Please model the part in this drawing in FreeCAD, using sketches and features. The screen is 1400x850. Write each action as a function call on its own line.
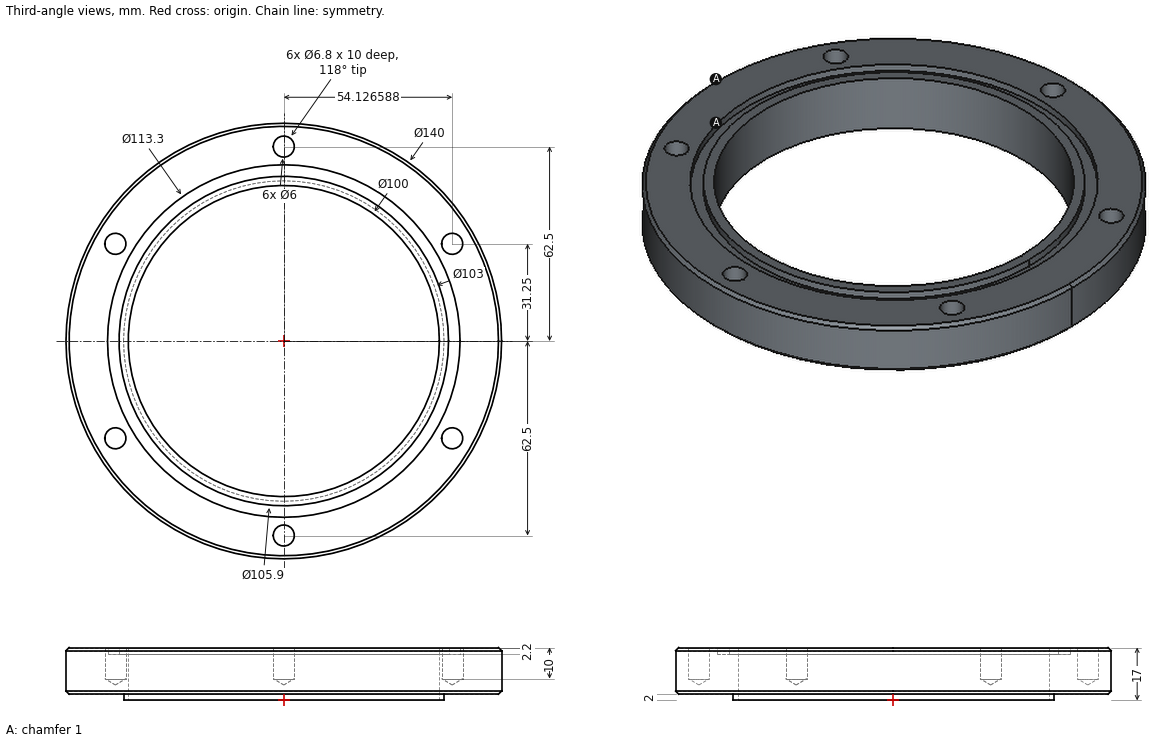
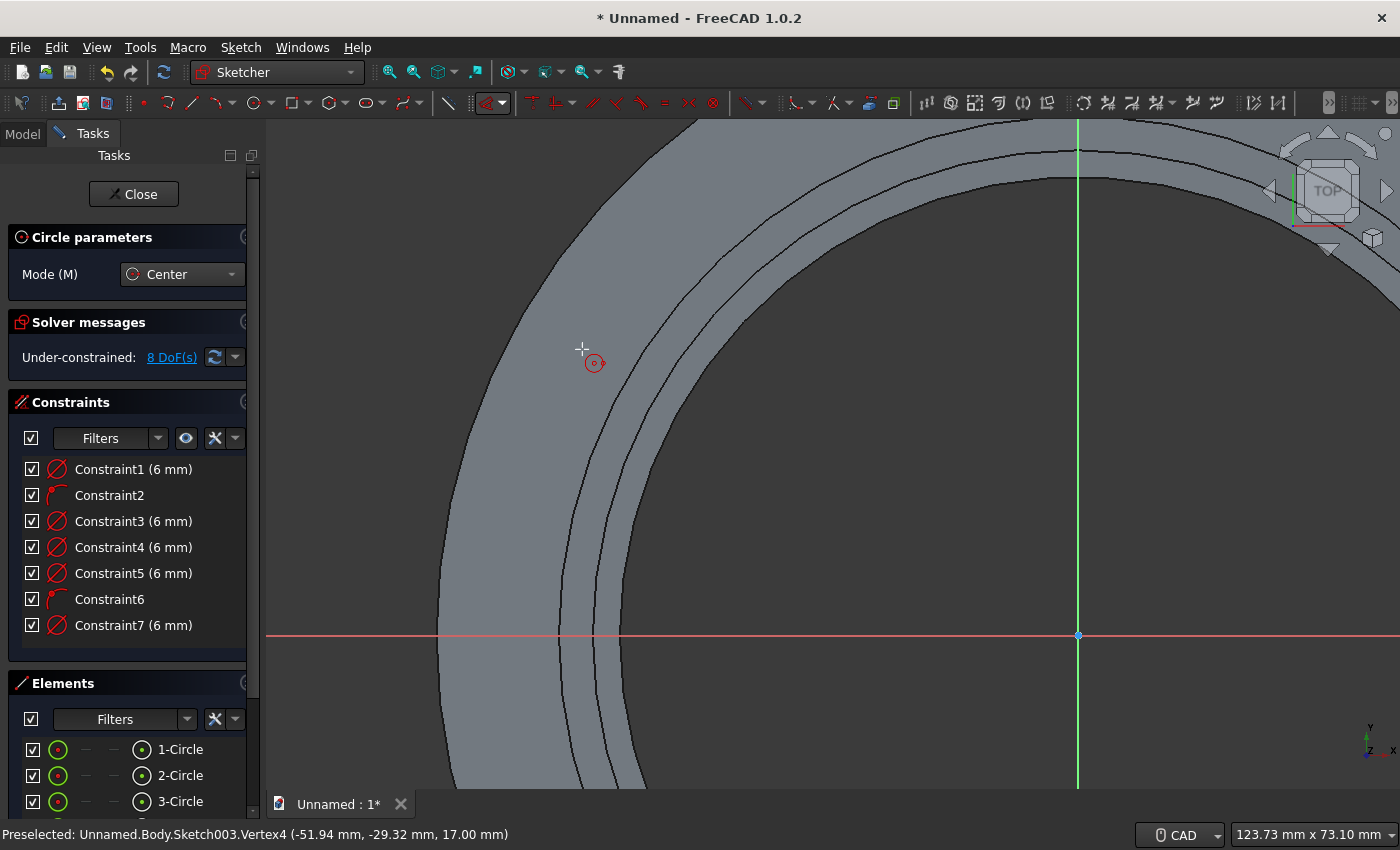
click(582, 349)
move(601, 330)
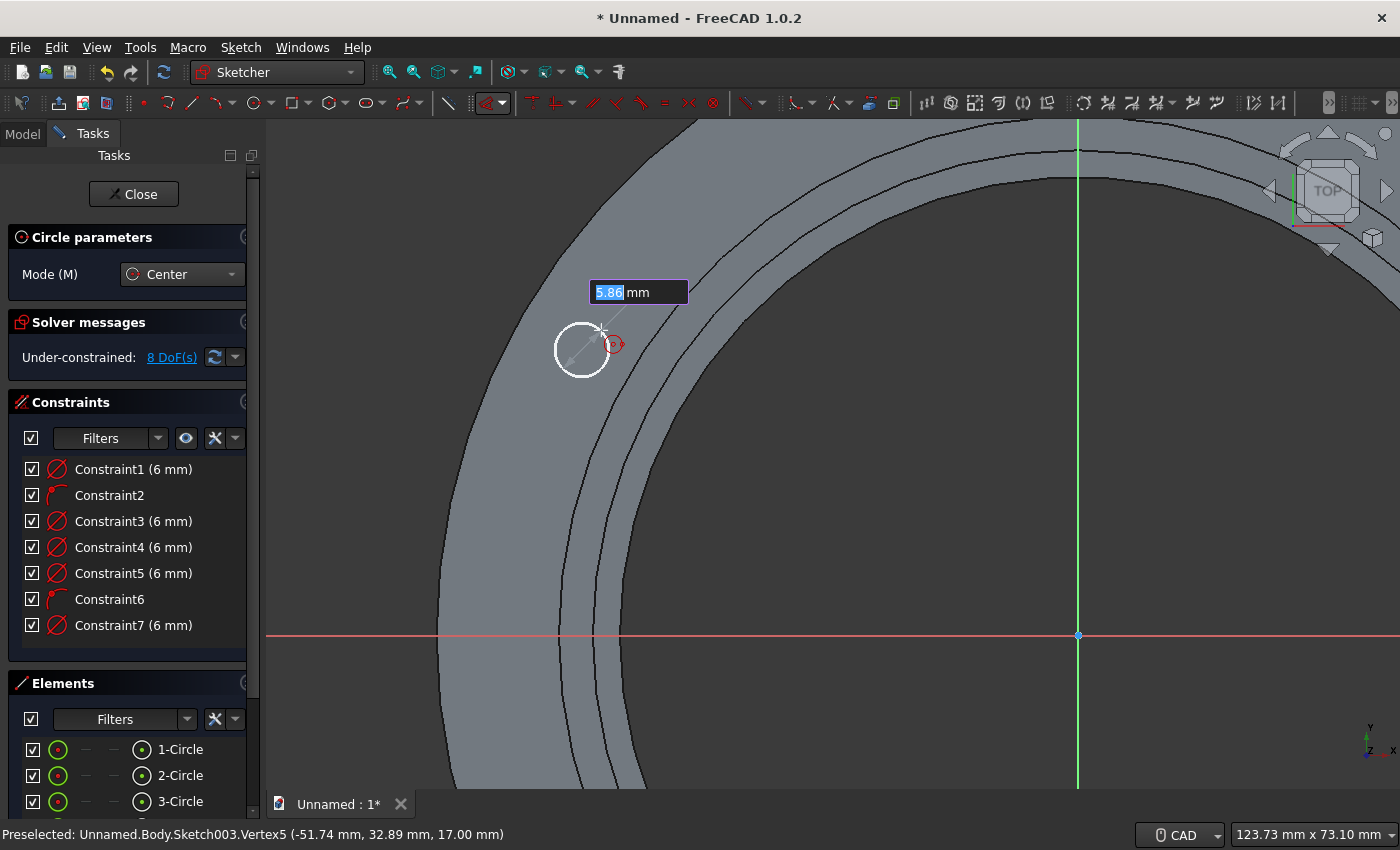
text(6)
key(Return)
key(Escape)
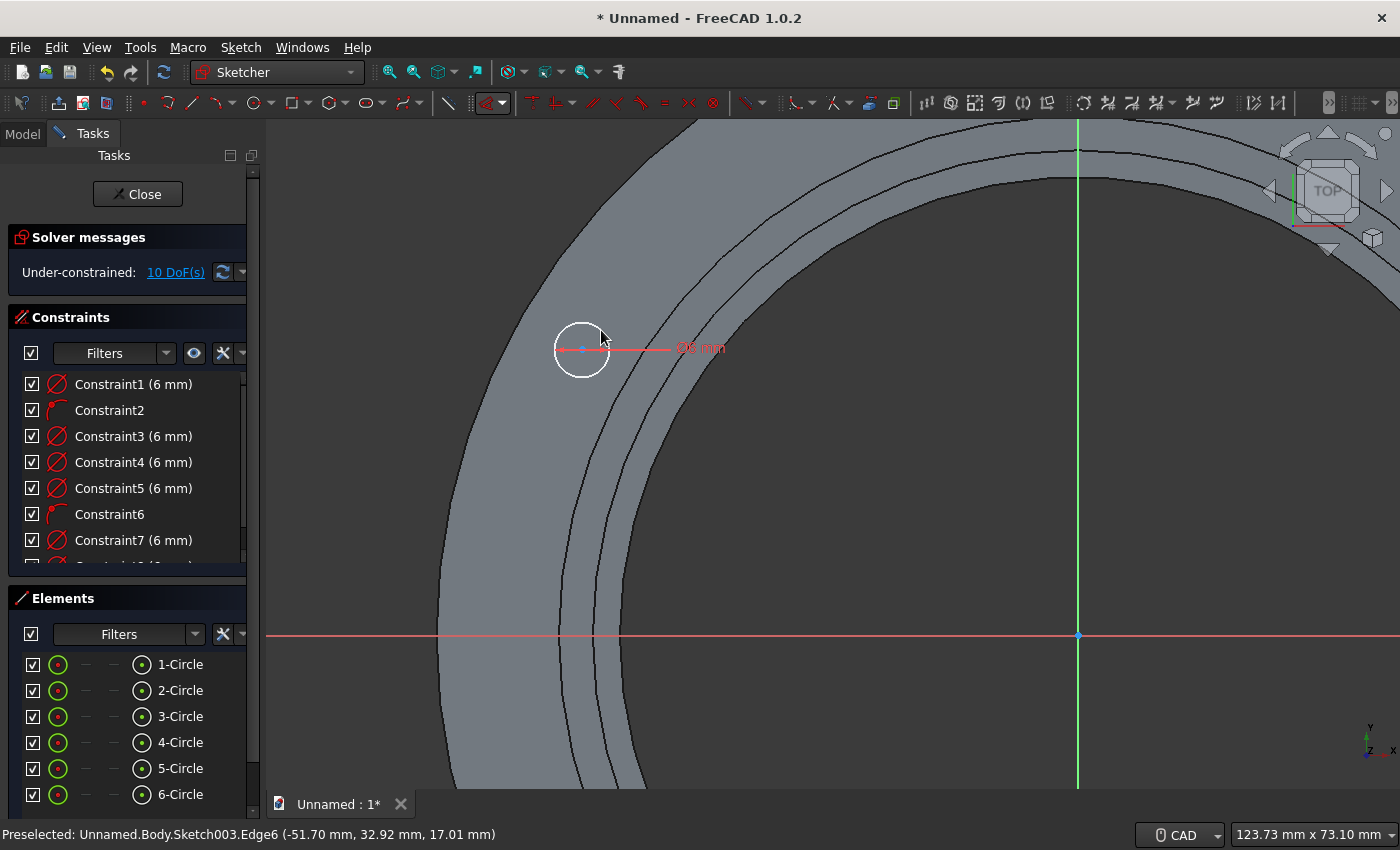
scroll(582, 348, down, 5)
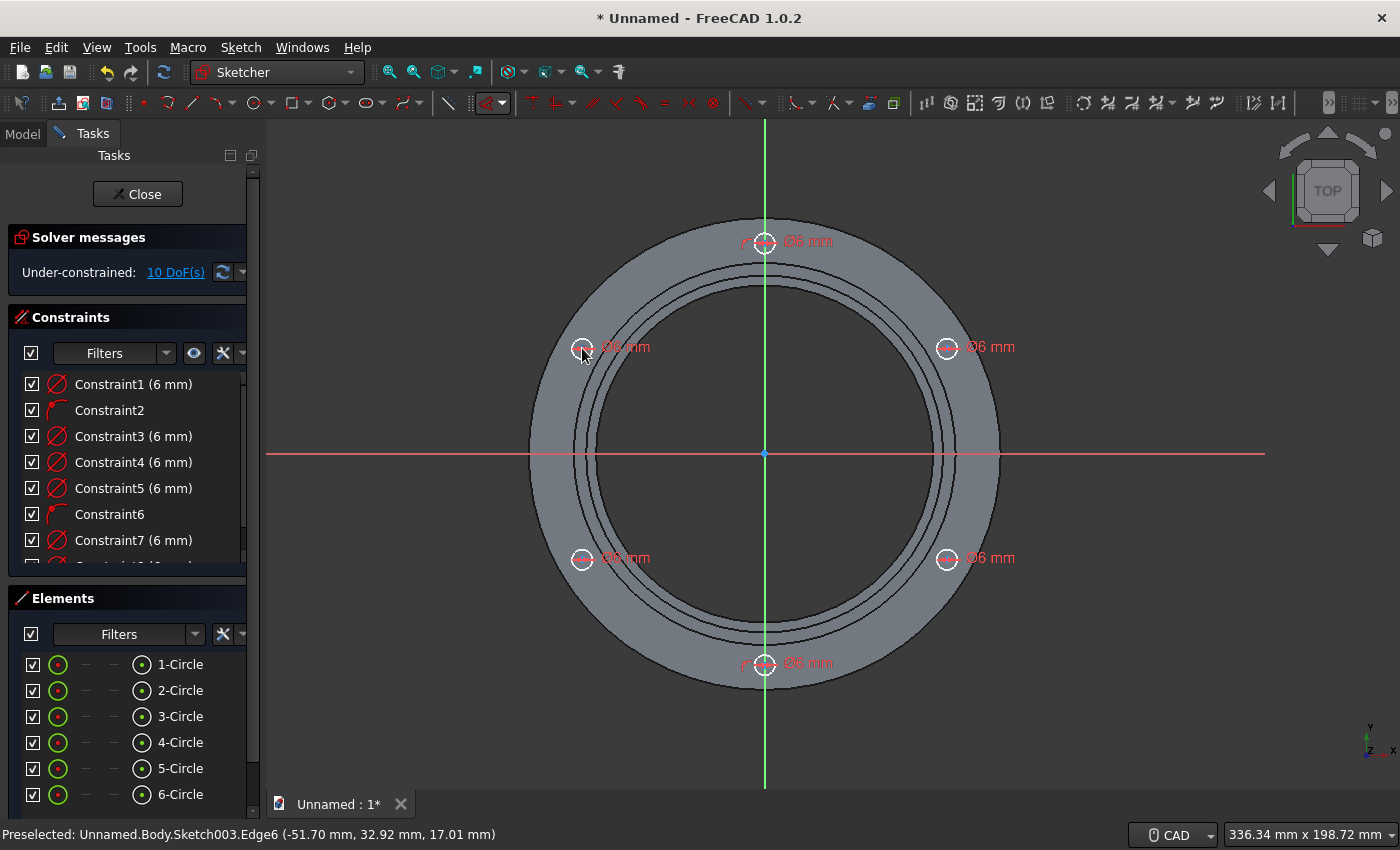
click(947, 349)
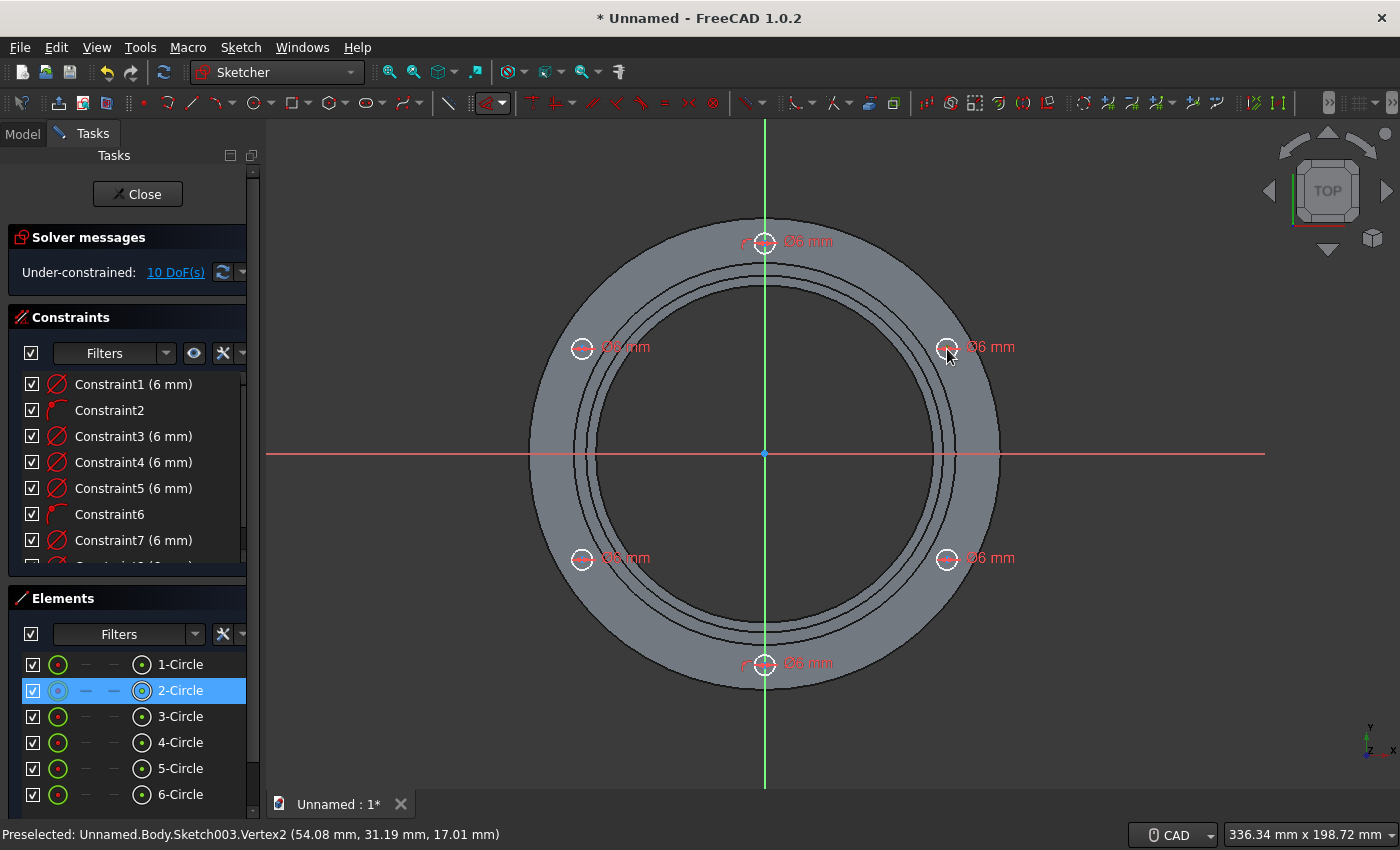
click(947, 560)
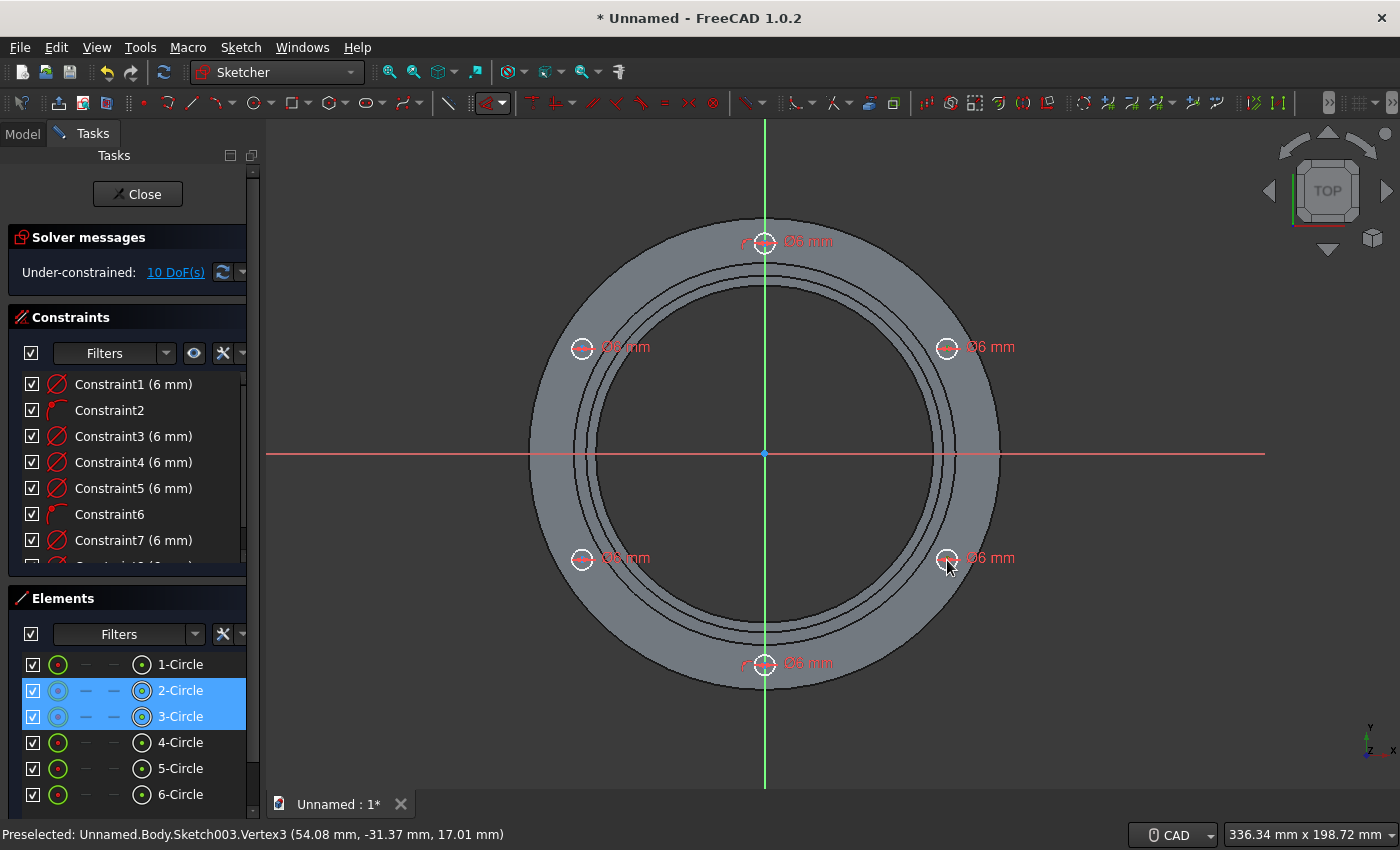
click(361, 454)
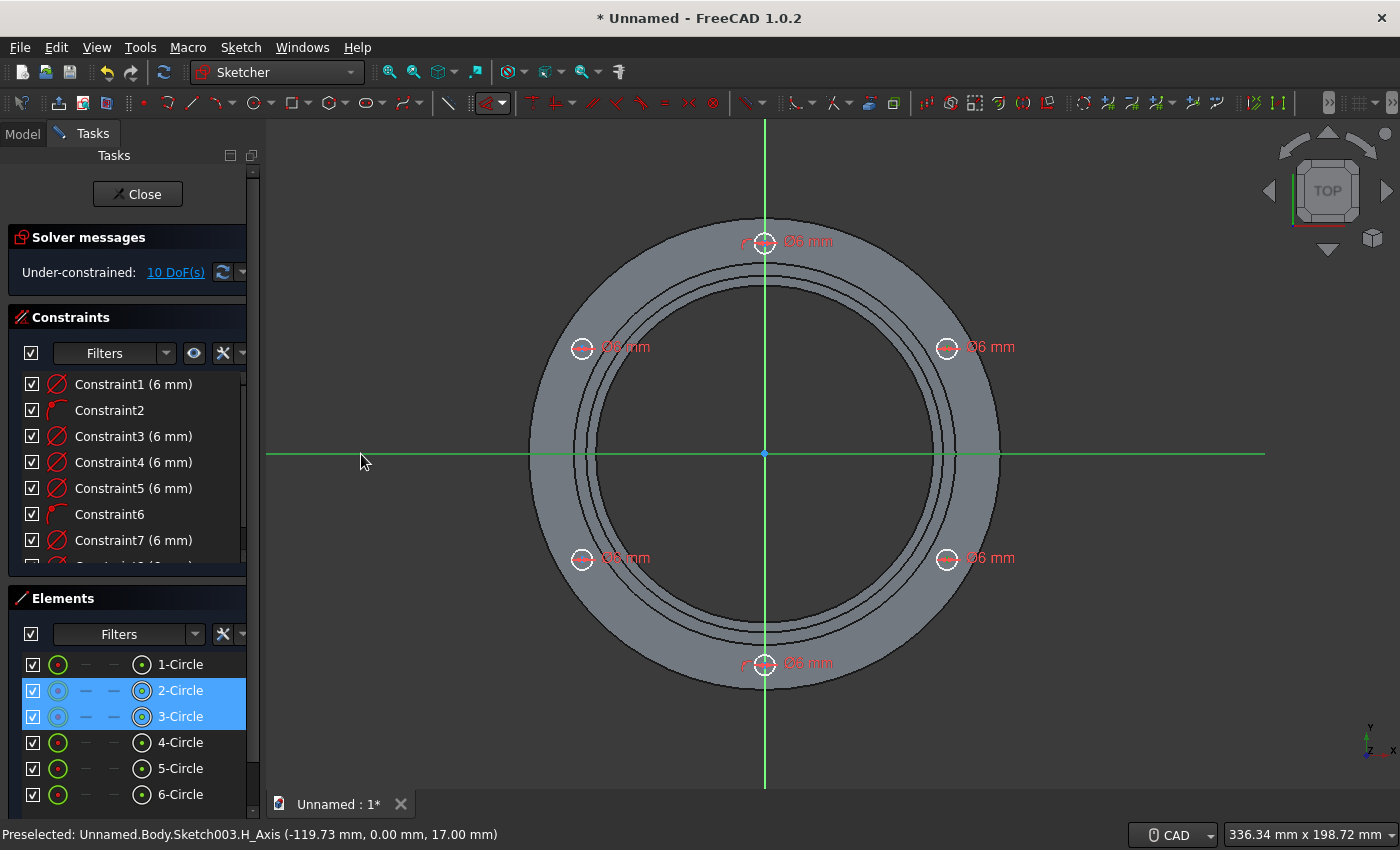
key(s)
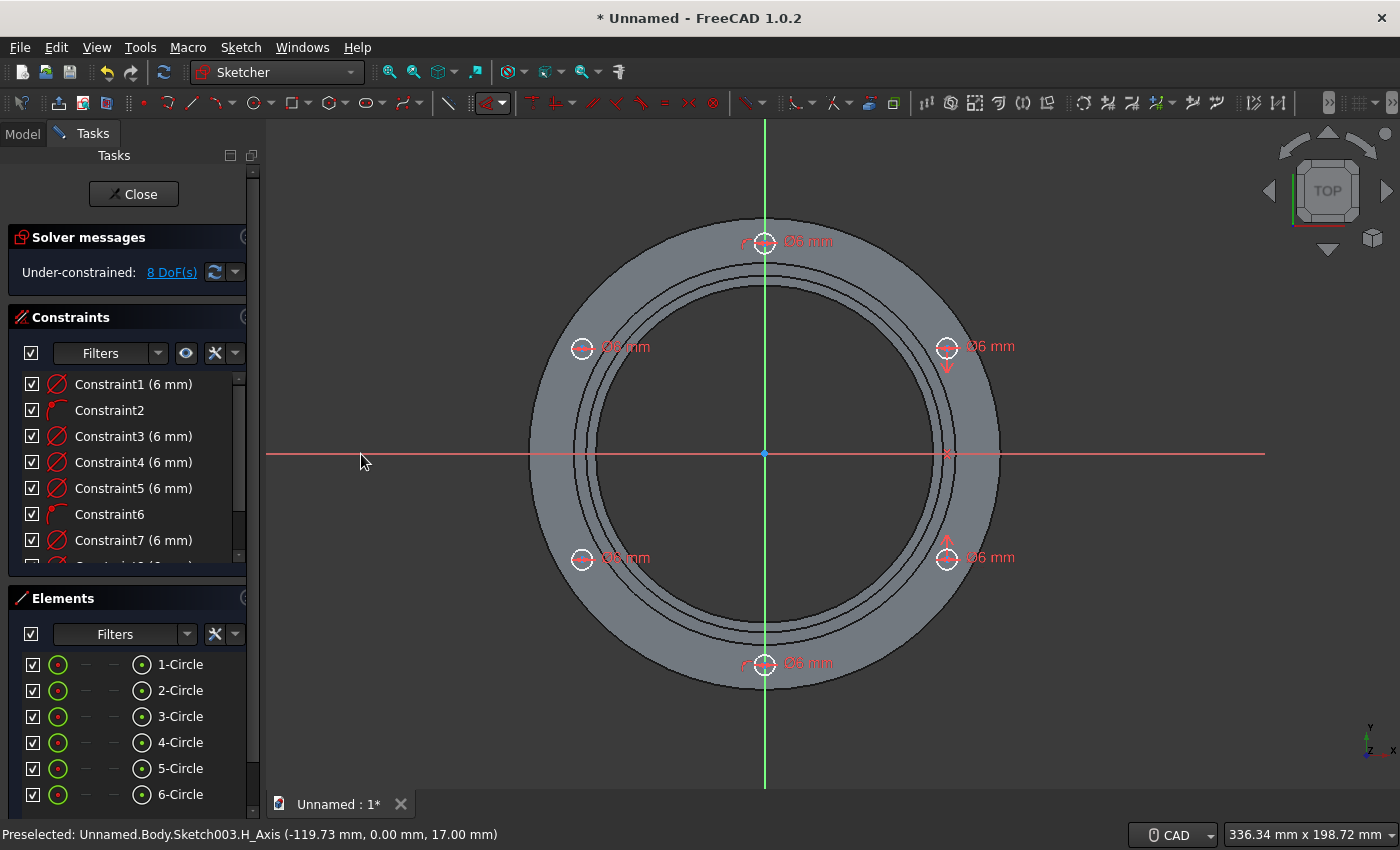
click(947, 560)